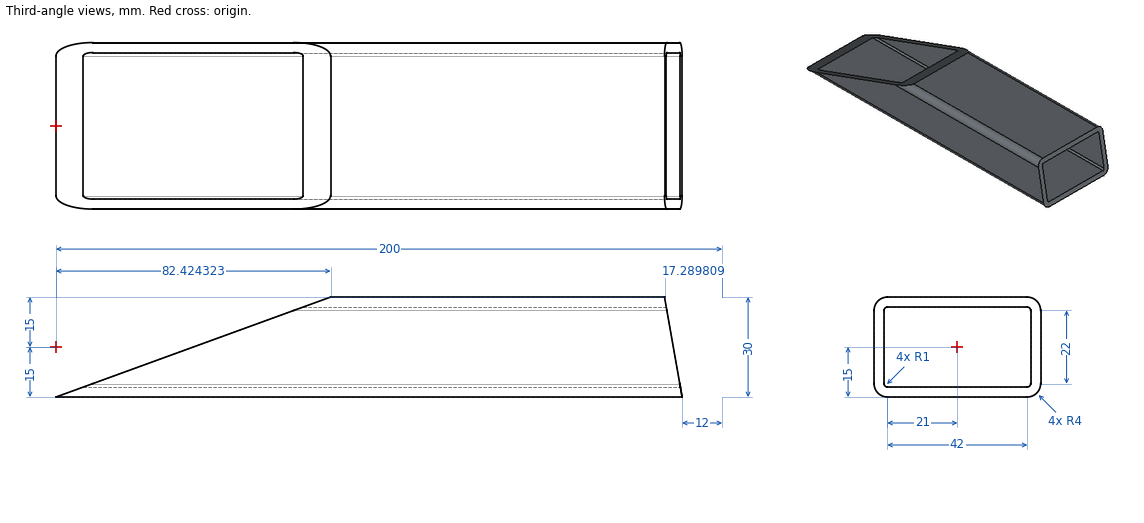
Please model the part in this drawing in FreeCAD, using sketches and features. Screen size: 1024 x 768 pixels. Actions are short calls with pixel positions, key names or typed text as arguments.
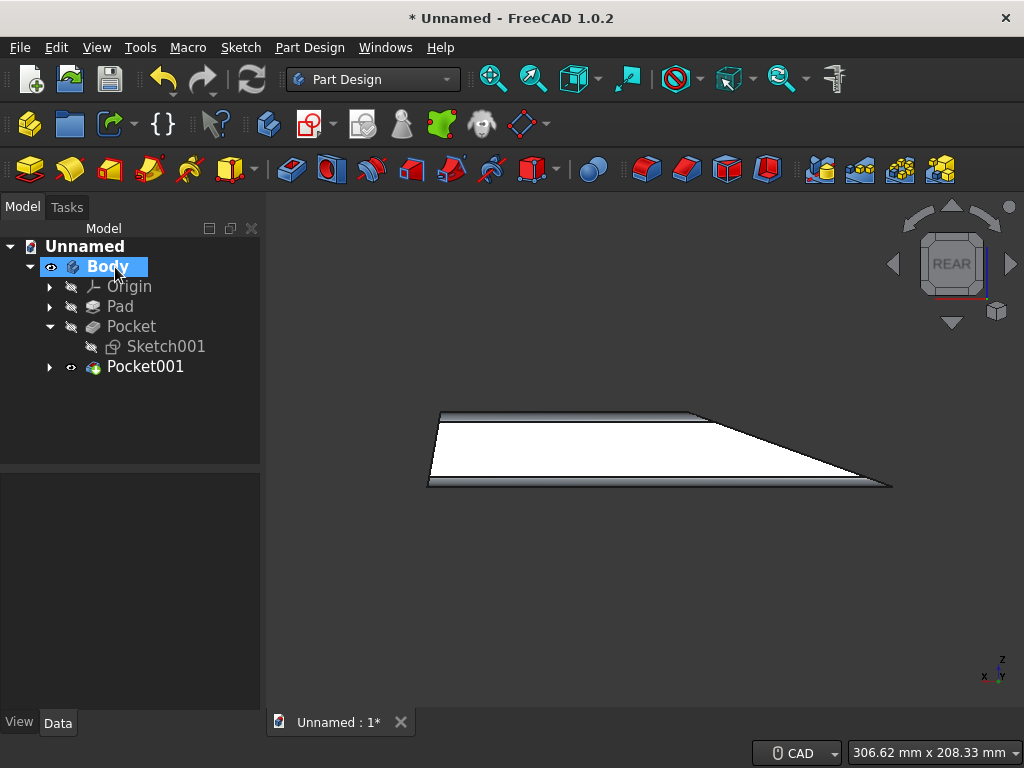
key(0)